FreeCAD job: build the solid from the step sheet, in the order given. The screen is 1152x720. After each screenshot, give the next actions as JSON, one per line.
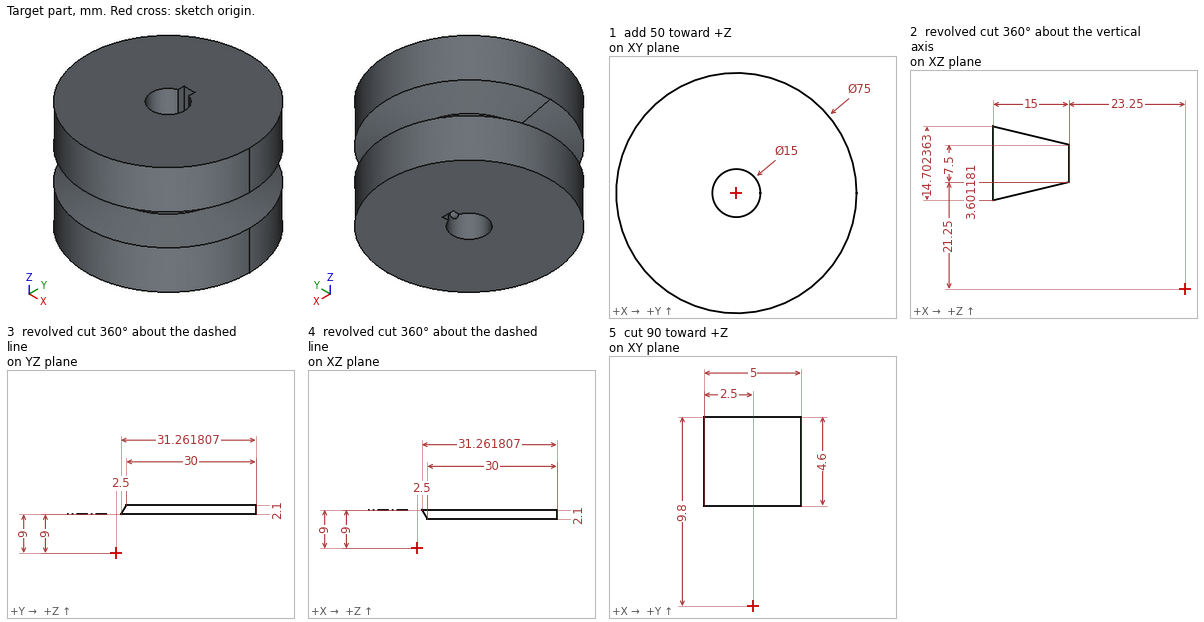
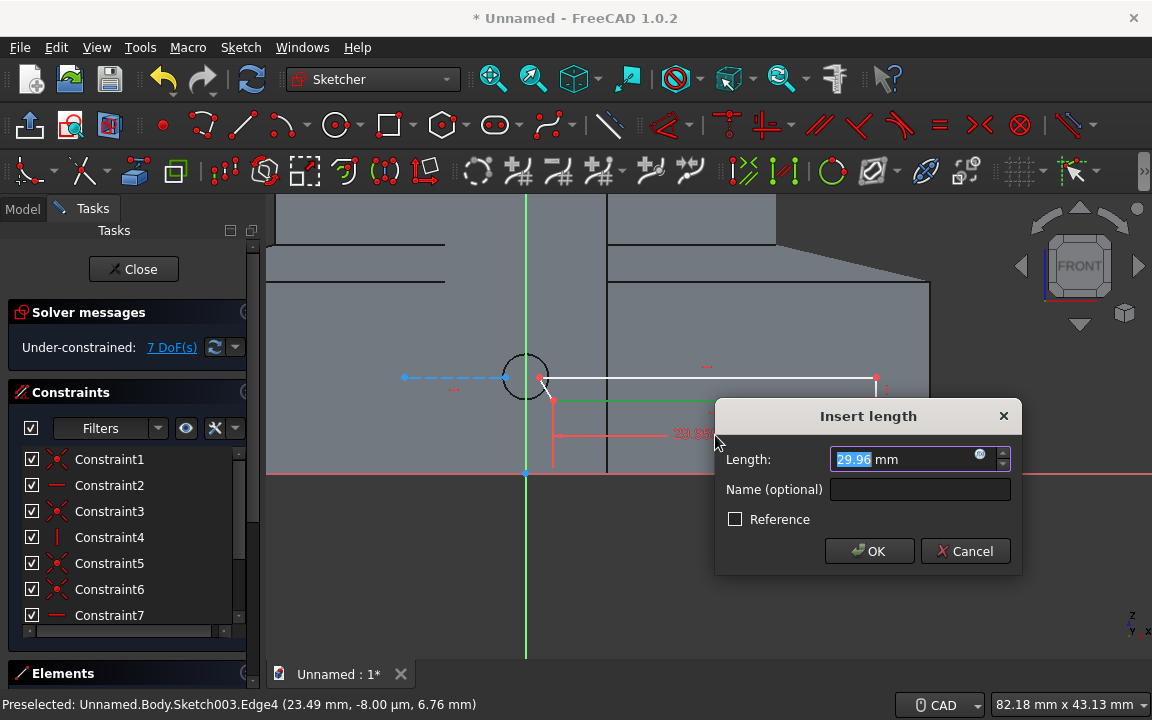
{"action": "type", "text": "30"}
{"action": "key", "text": "Return"}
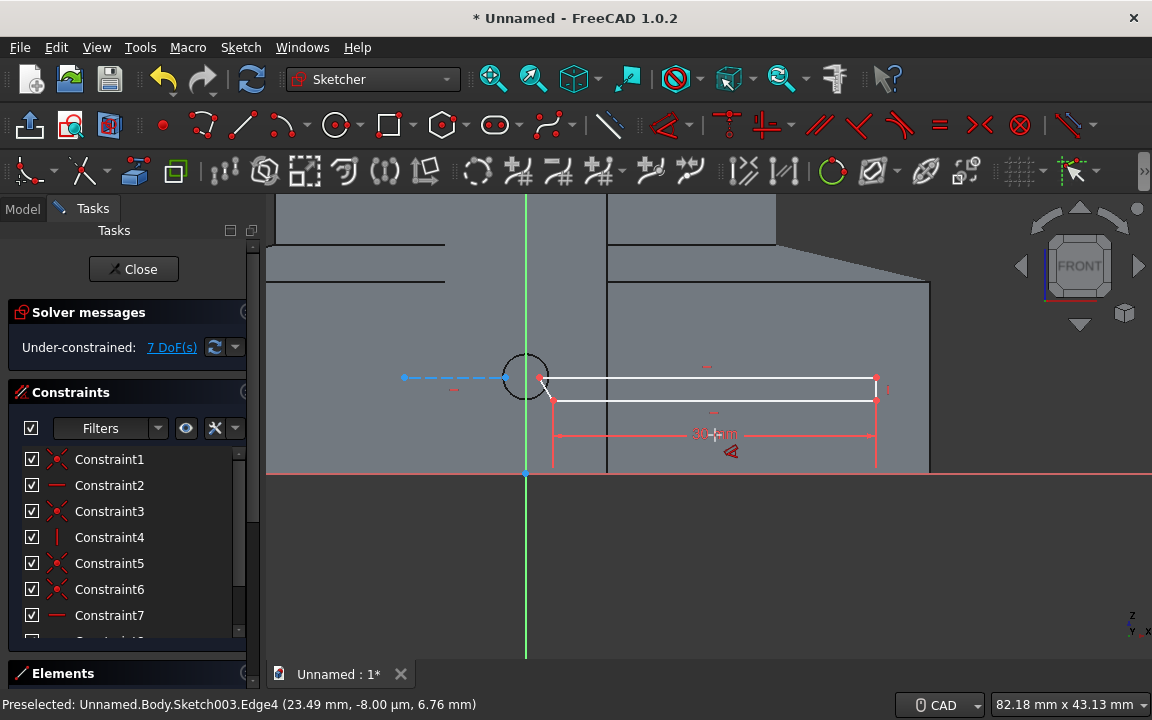
{"action": "left_click", "coordinate": [539, 378]}
{"action": "left_click", "coordinate": [492, 426]}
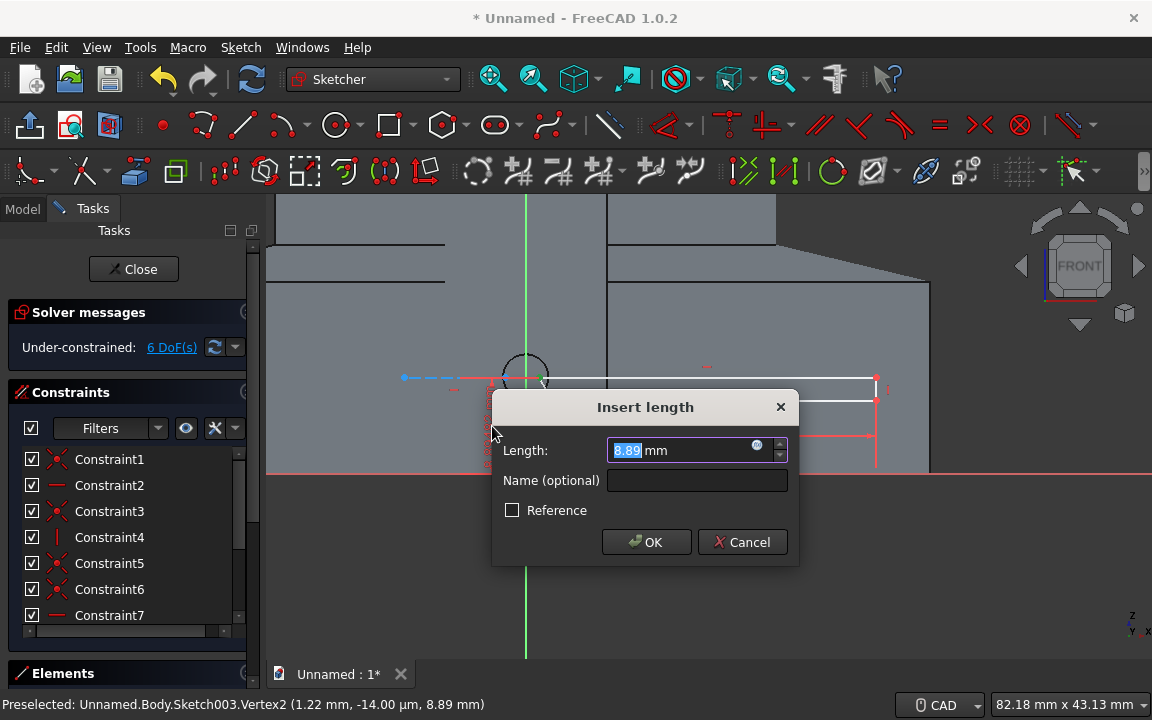
{"action": "type", "text": "9"}
{"action": "key", "text": "Return"}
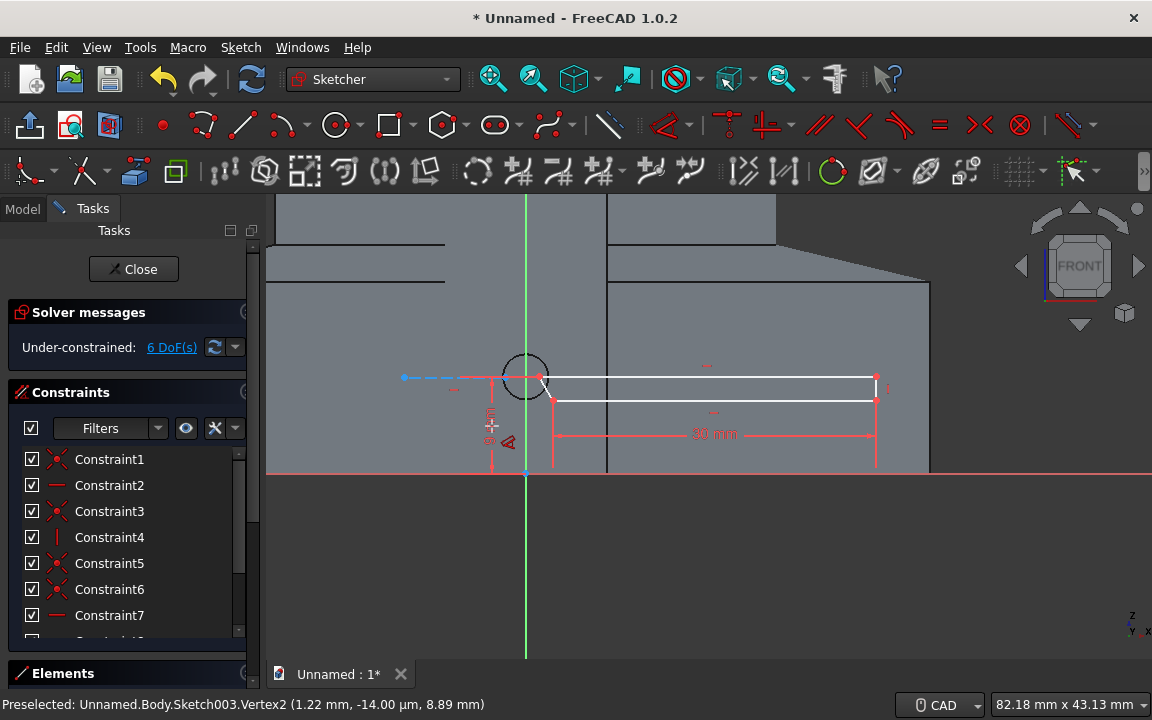
{"action": "left_click", "coordinate": [505, 378]}
{"action": "left_click", "coordinate": [471, 404]}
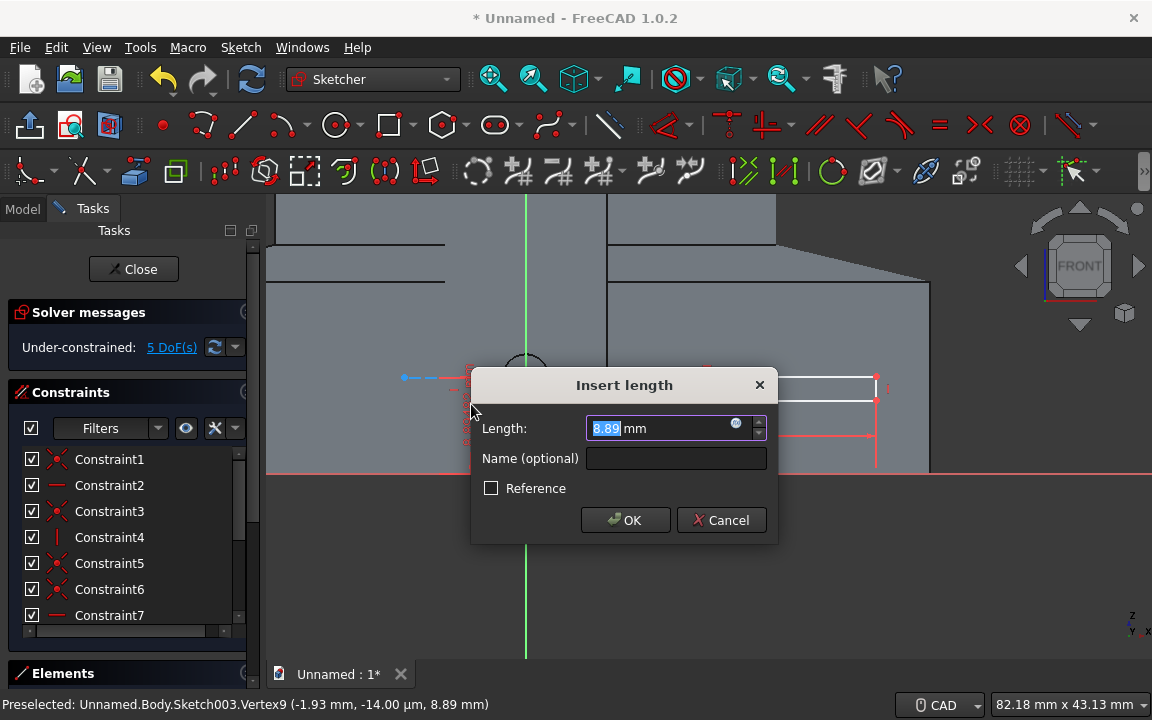
{"action": "type", "text": "9"}
{"action": "key", "text": "Return"}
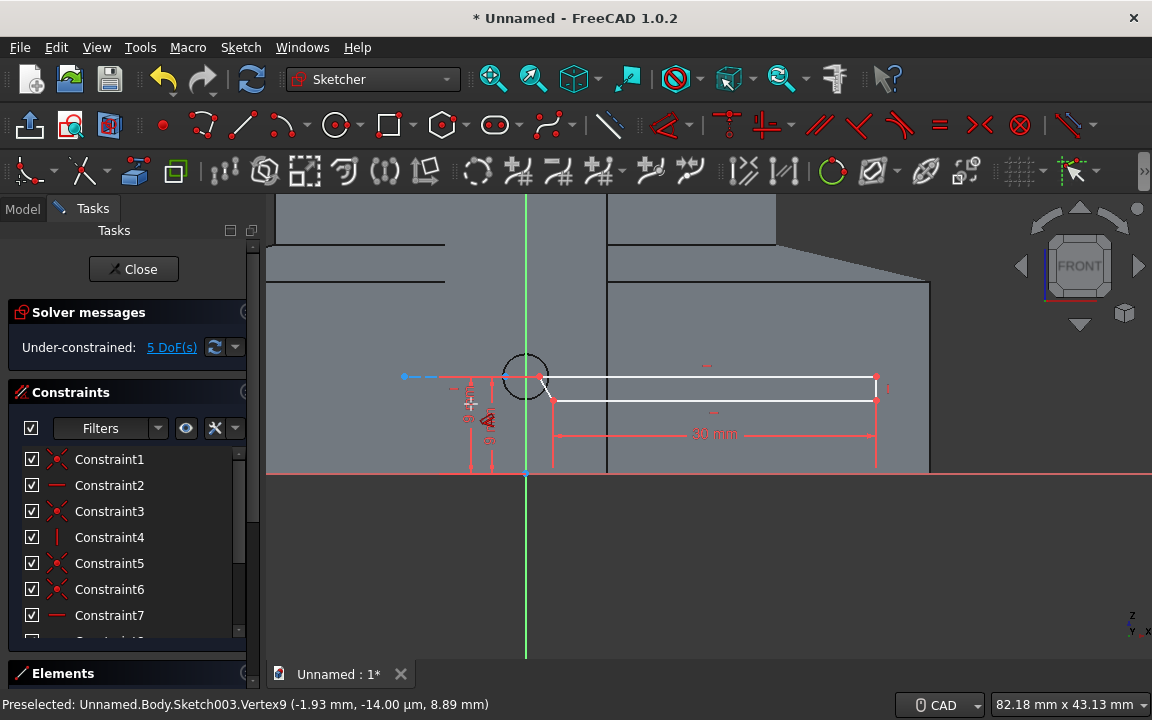
{"action": "scroll", "coordinate": [876, 387], "scroll_direction": "up", "scroll_amount": 3}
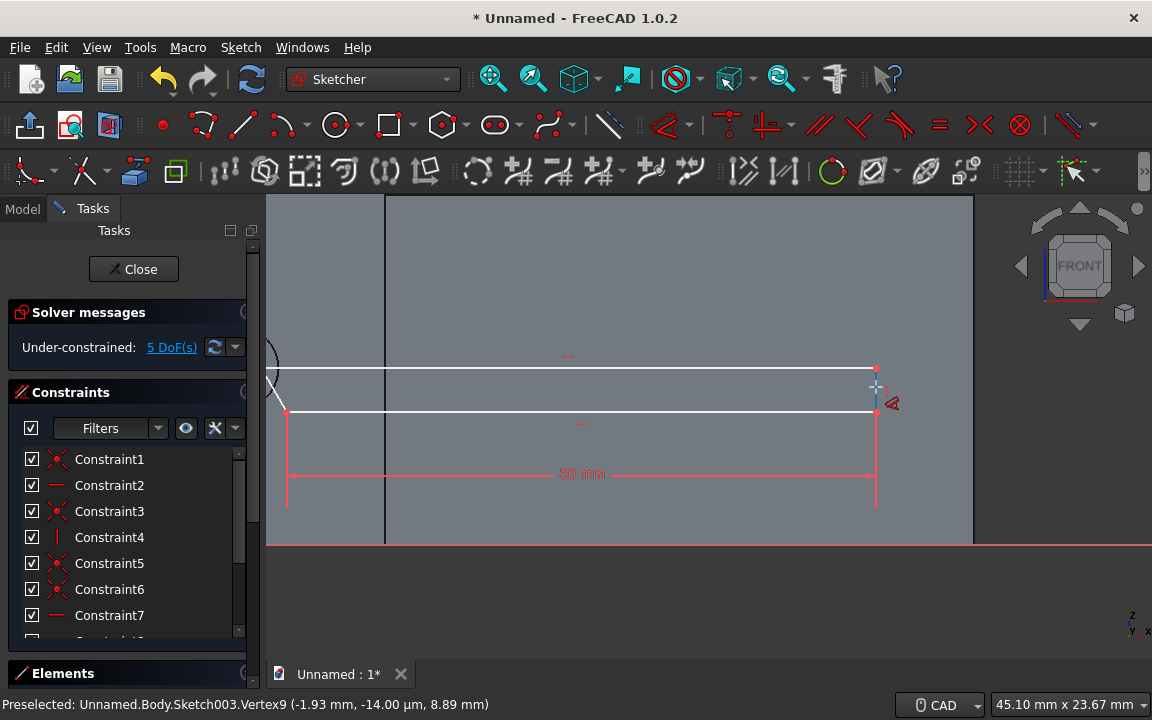
{"action": "left_click", "coordinate": [876, 386]}
{"action": "left_click", "coordinate": [910, 390]}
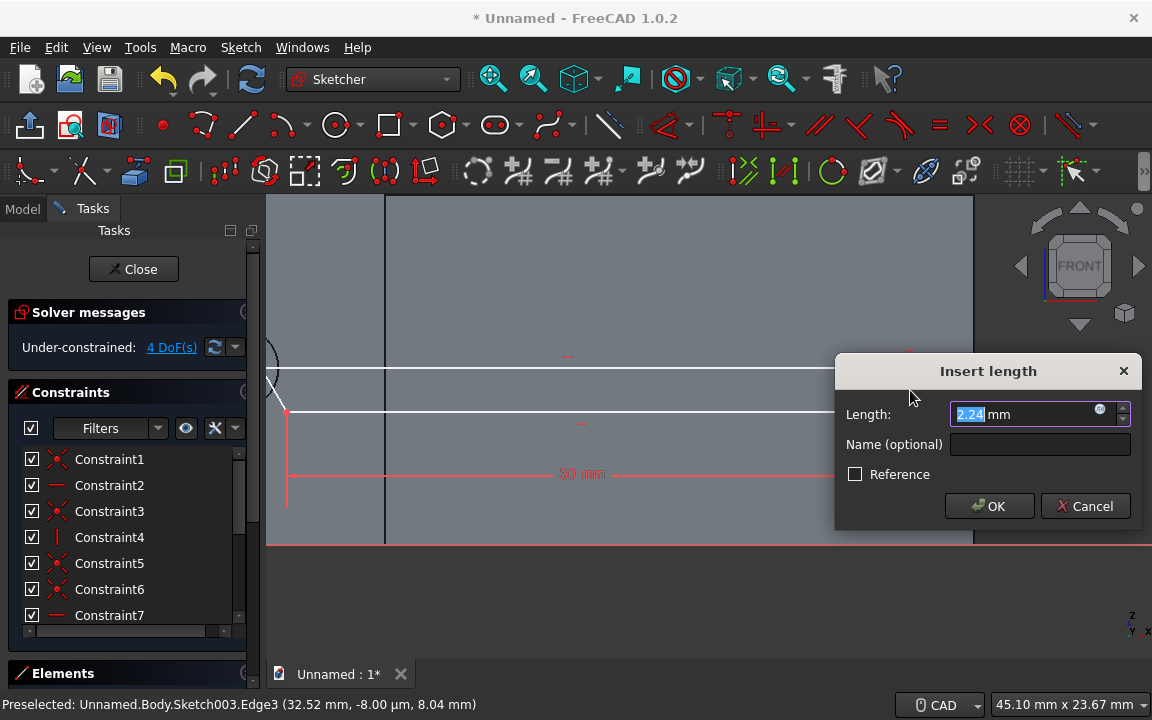
{"action": "type", "text": "2.1"}
{"action": "key", "text": "Return"}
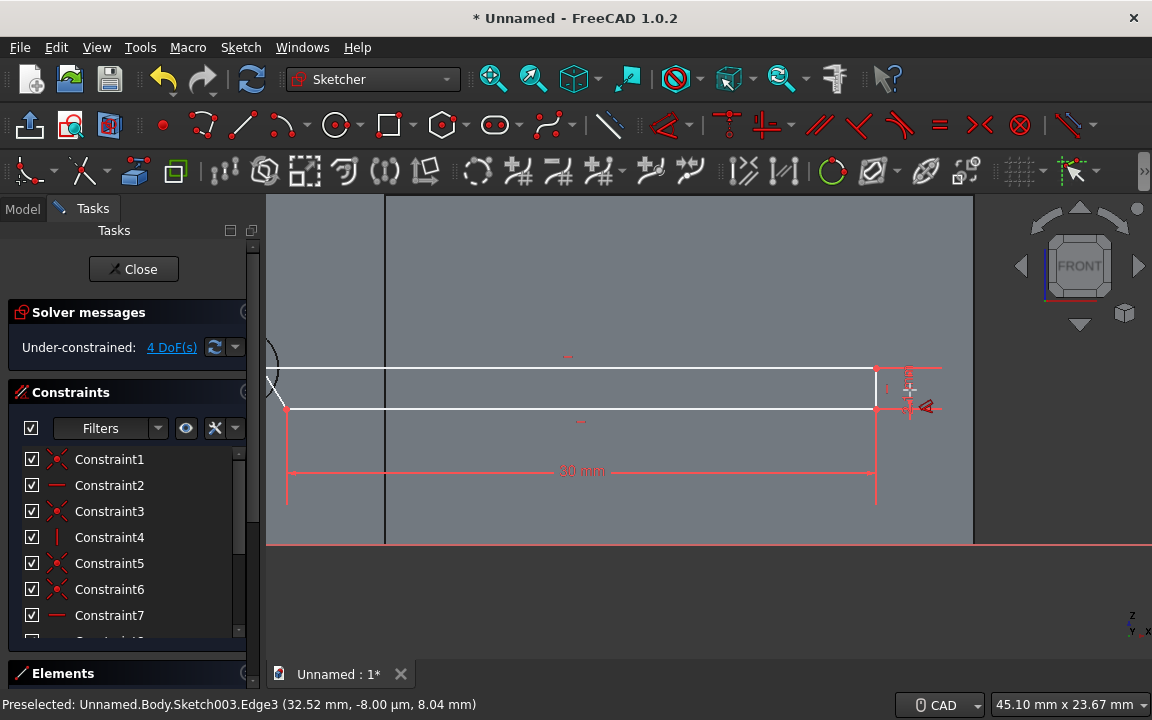
{"action": "scroll", "coordinate": [877, 390], "scroll_direction": "down", "scroll_amount": 3}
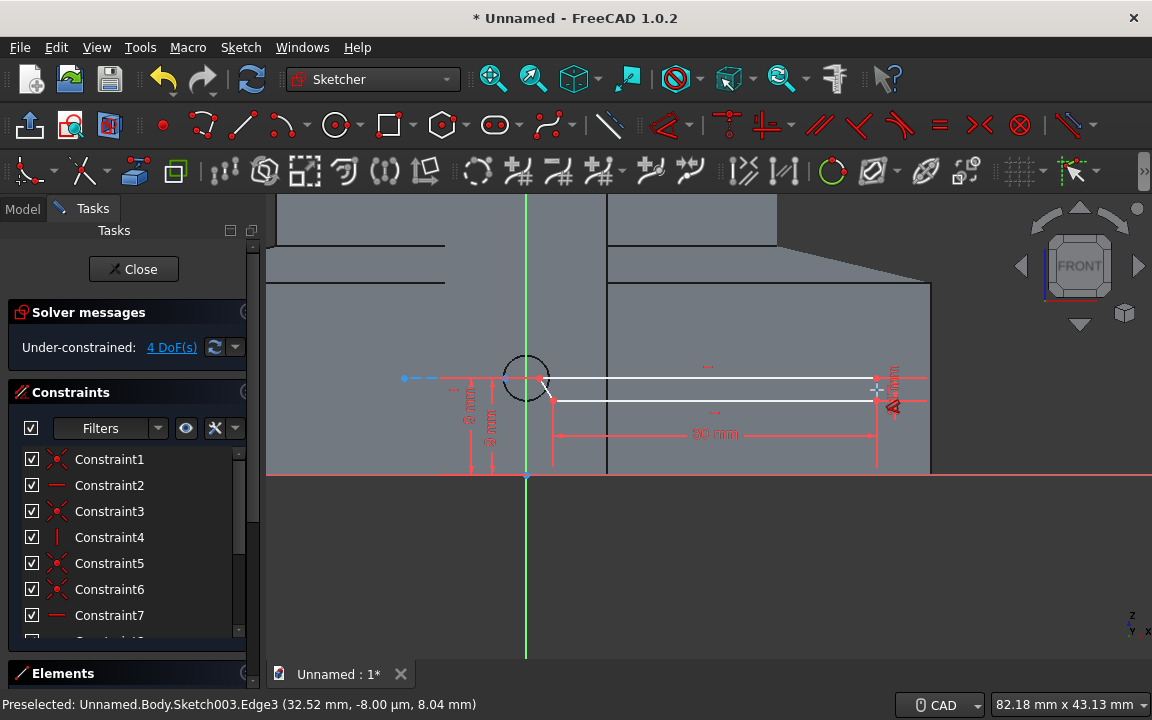
{"action": "scroll", "coordinate": [553, 401], "scroll_direction": "up", "scroll_amount": 2}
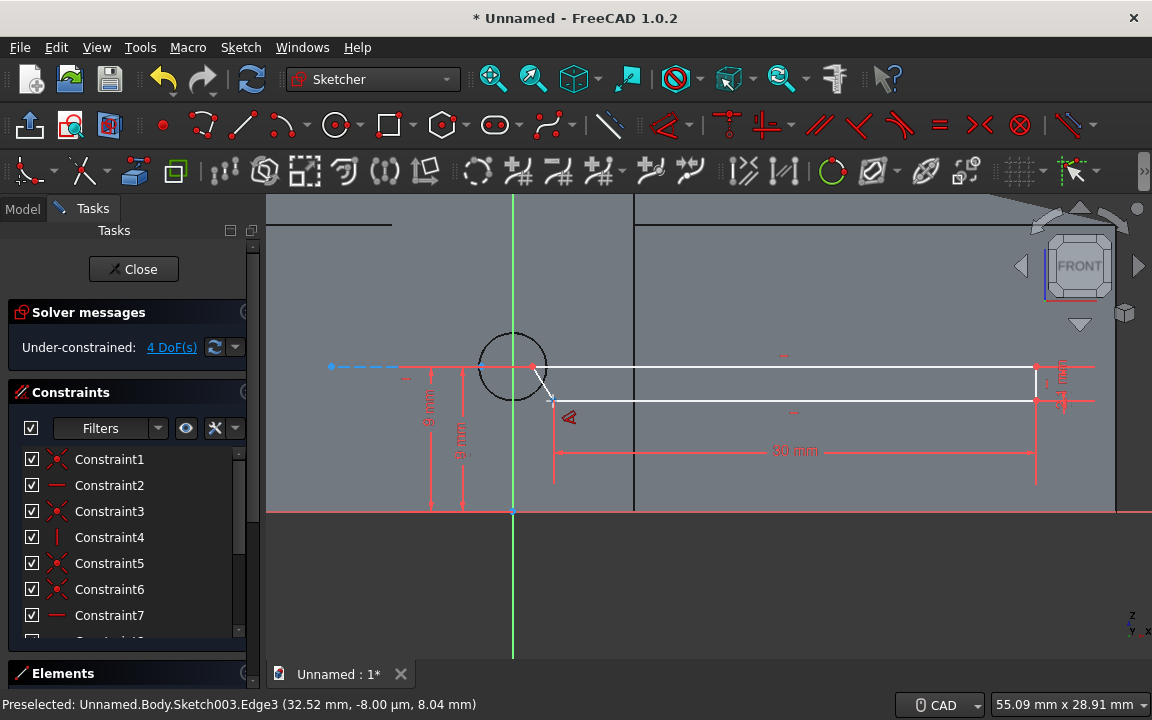
{"action": "left_click", "coordinate": [554, 401]}
{"action": "left_click", "coordinate": [533, 546]}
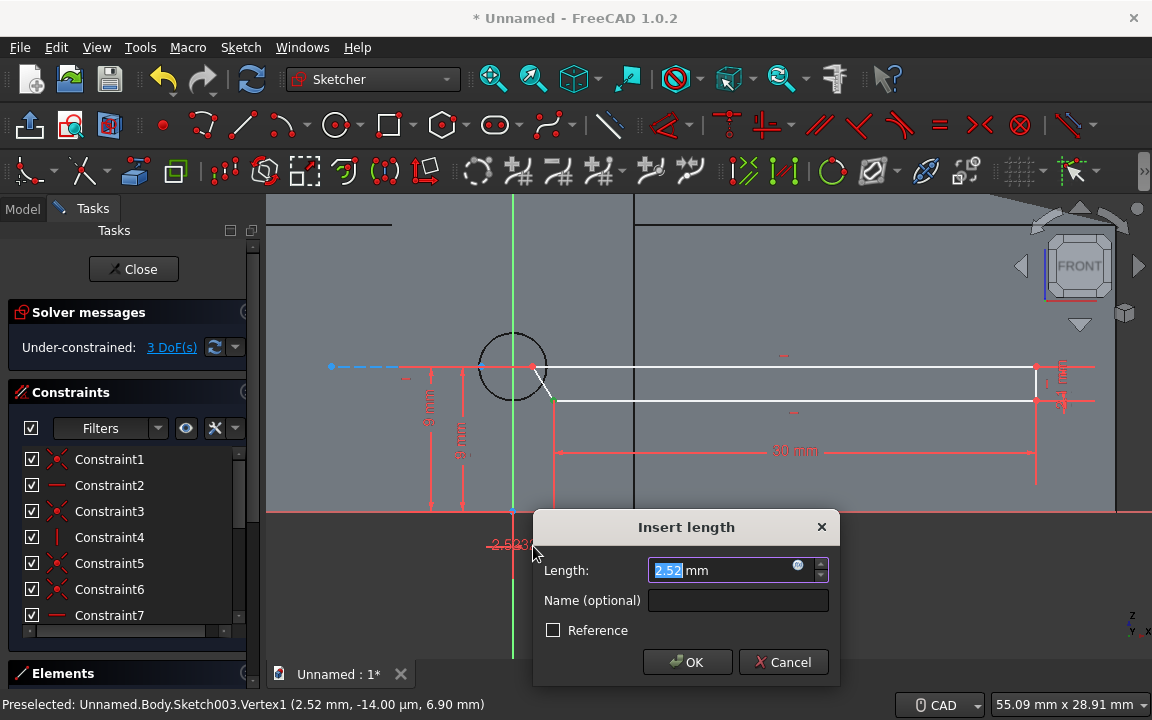
{"action": "type", "text": "2.5"}
{"action": "key", "text": "Return"}